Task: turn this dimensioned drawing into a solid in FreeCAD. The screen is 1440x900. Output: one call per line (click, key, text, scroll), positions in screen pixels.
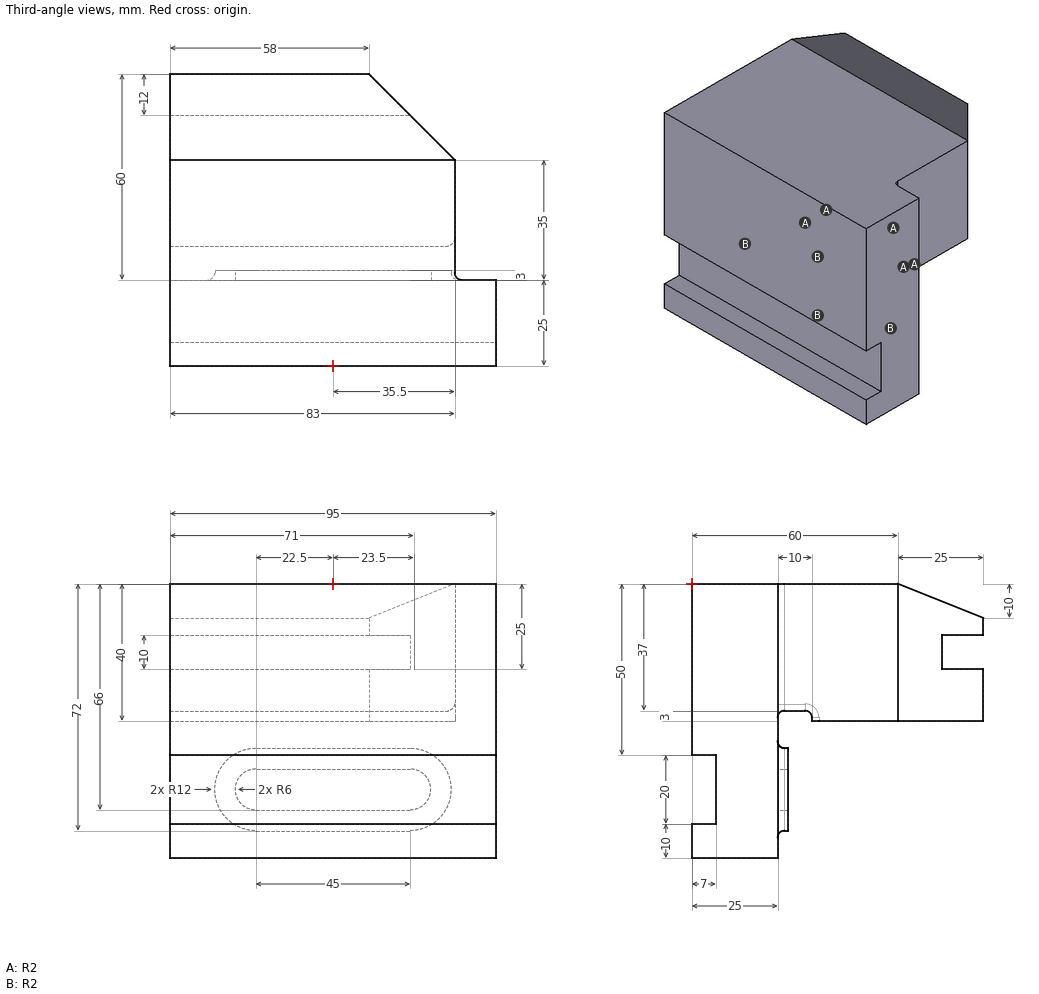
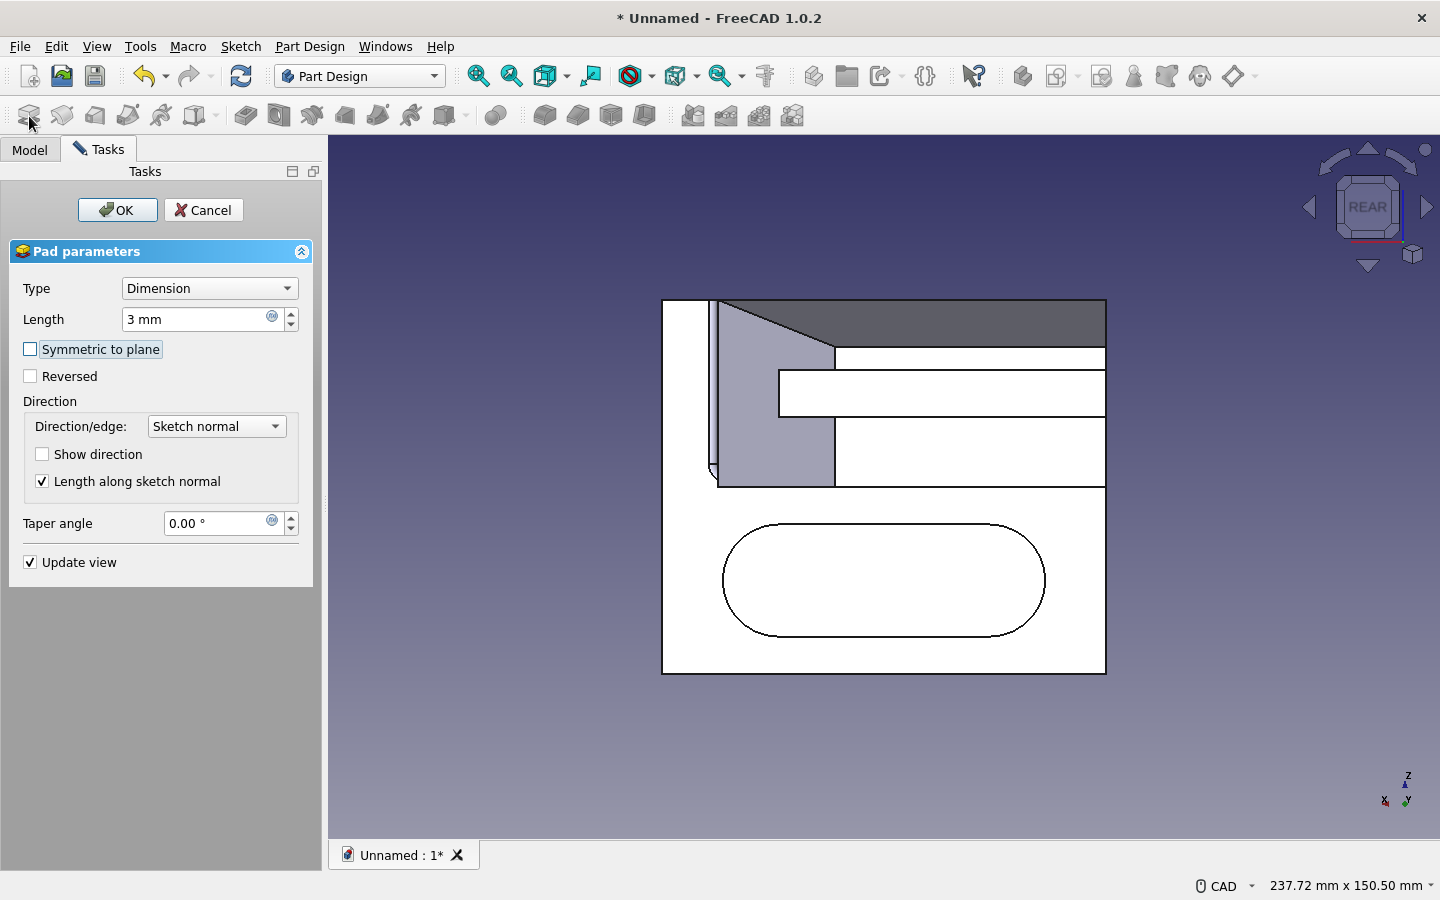
click(118, 210)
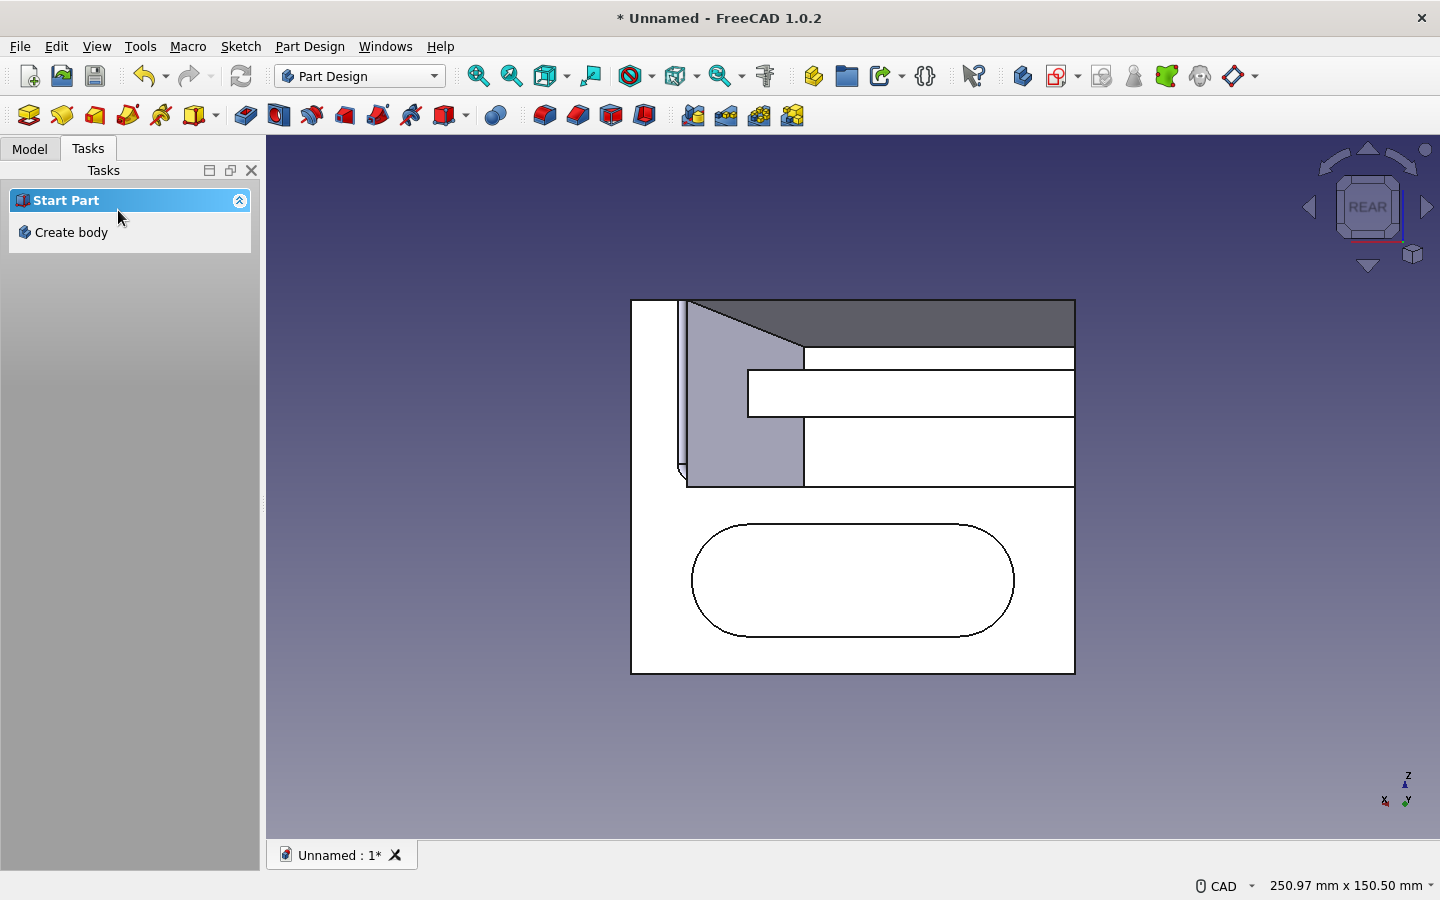
key(0)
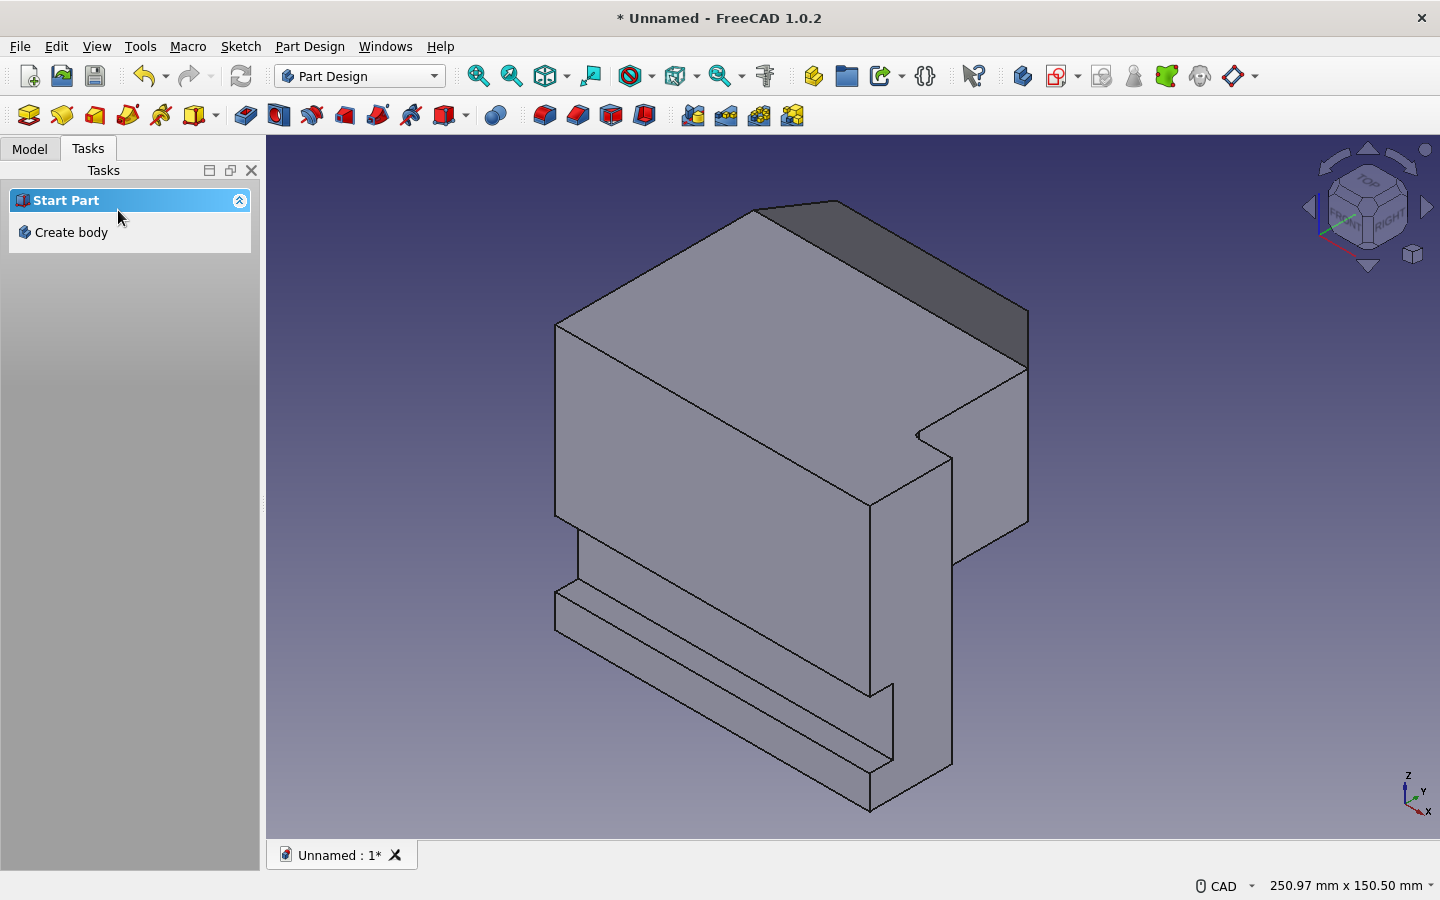
key(2)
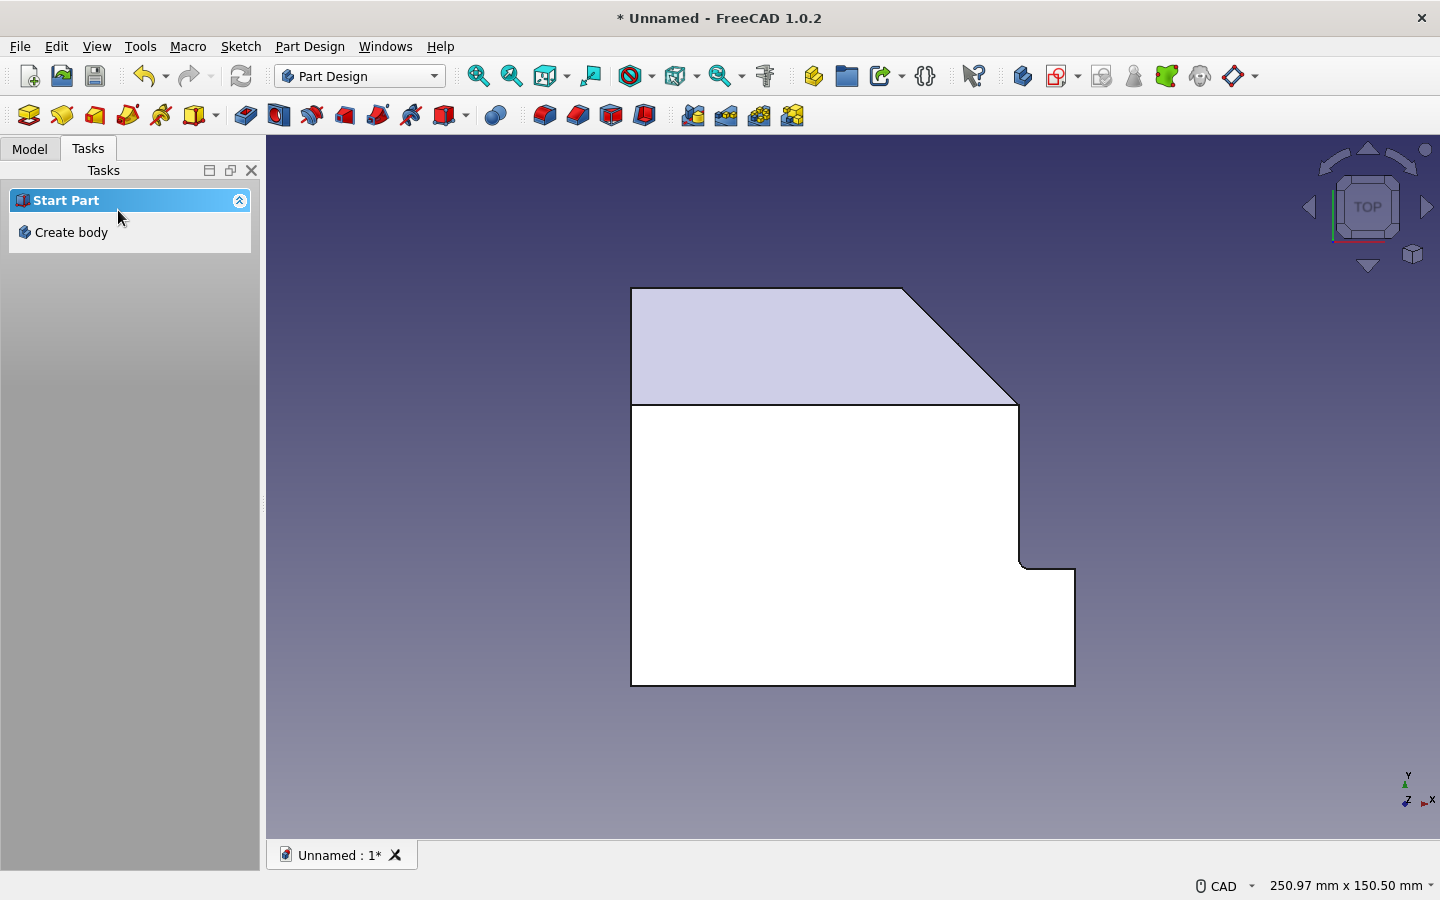
key(1)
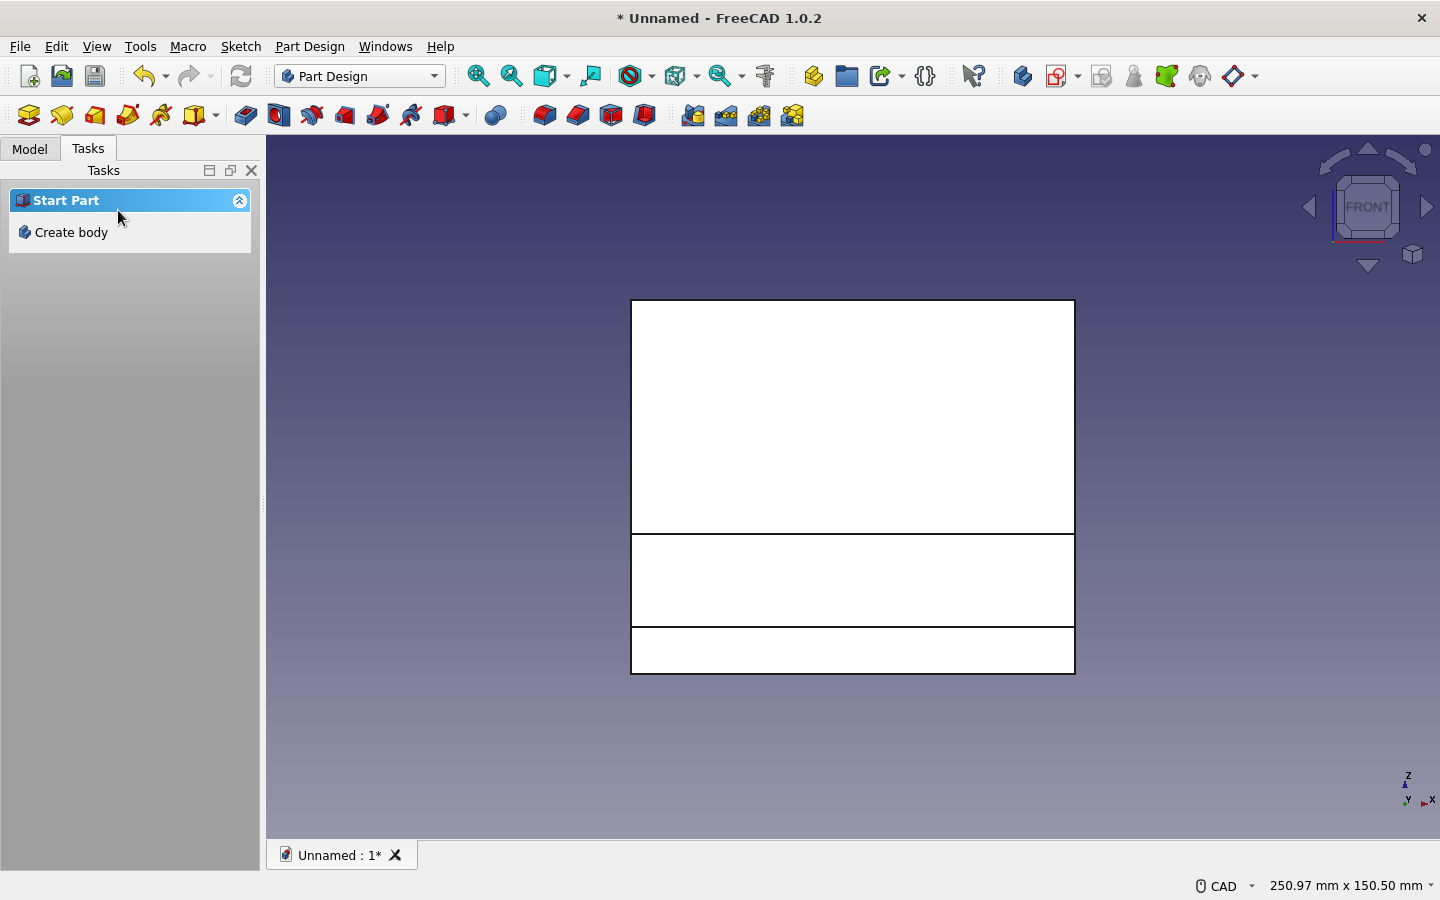
key(3)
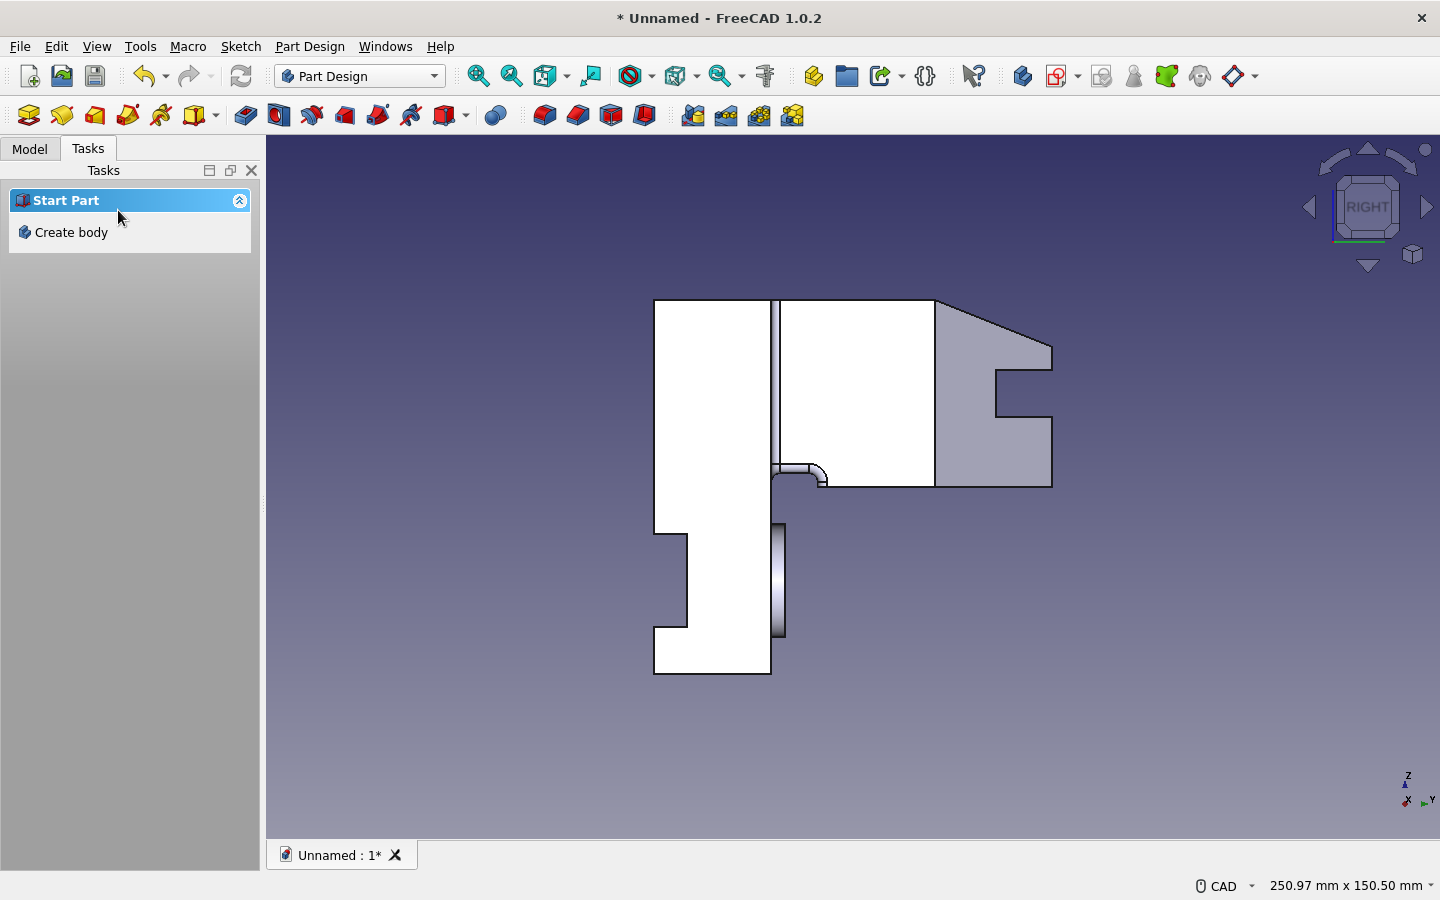
key(5)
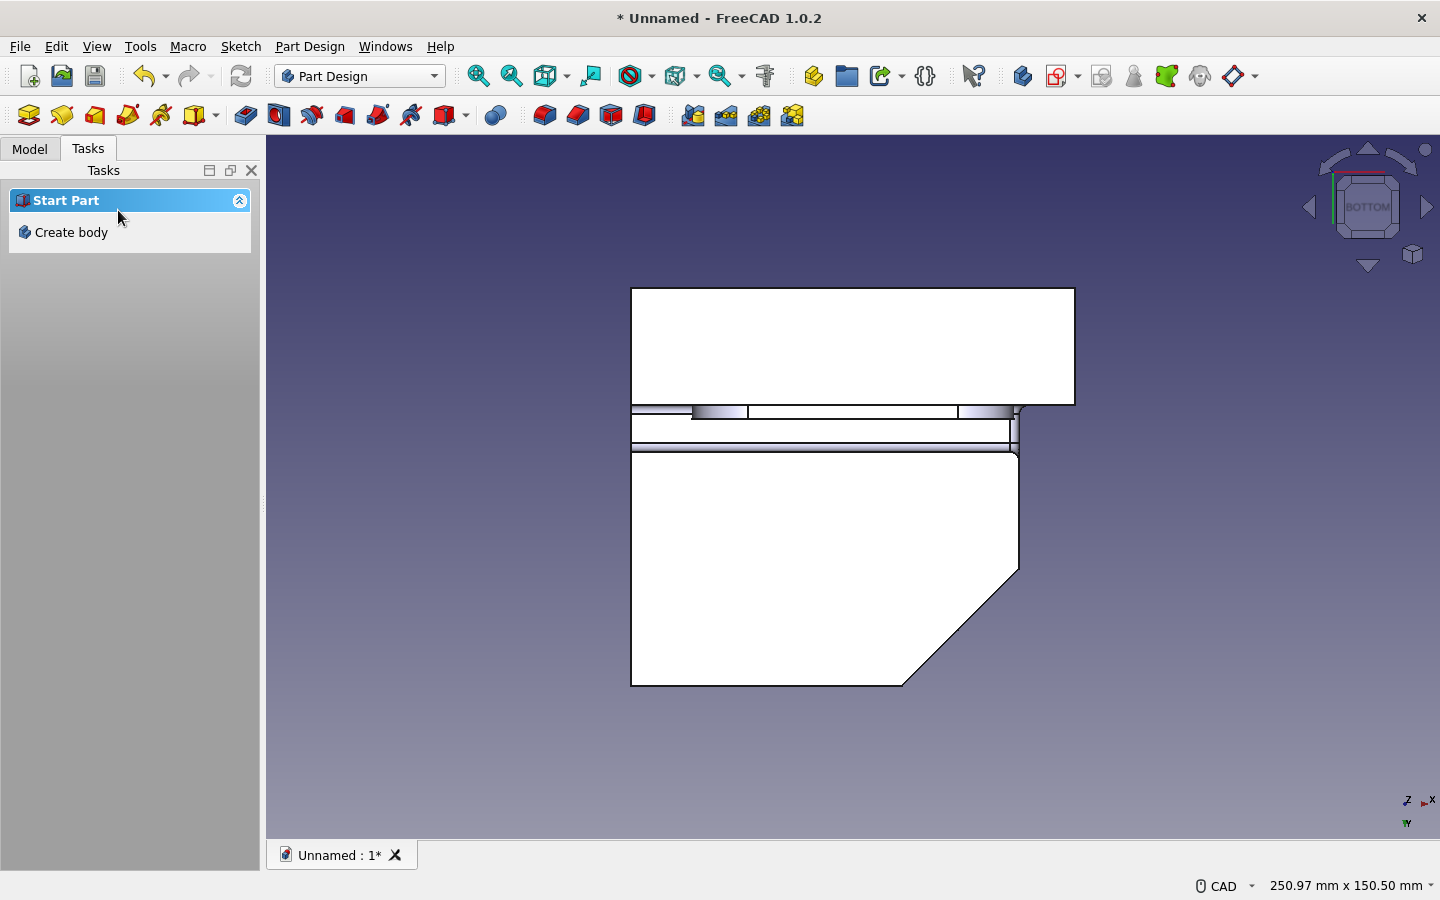
key(4)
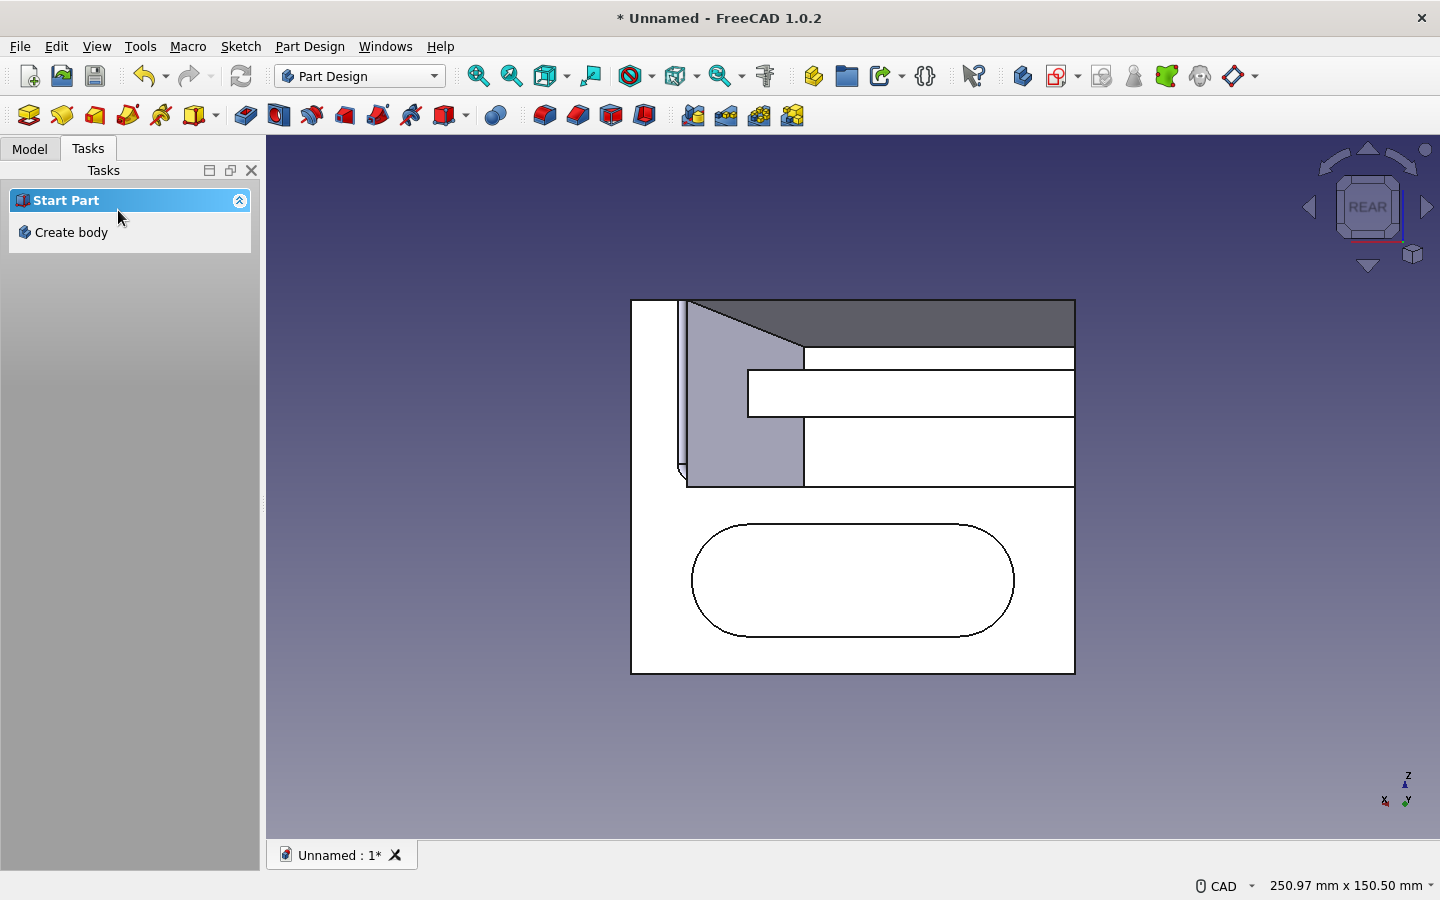
key(6)